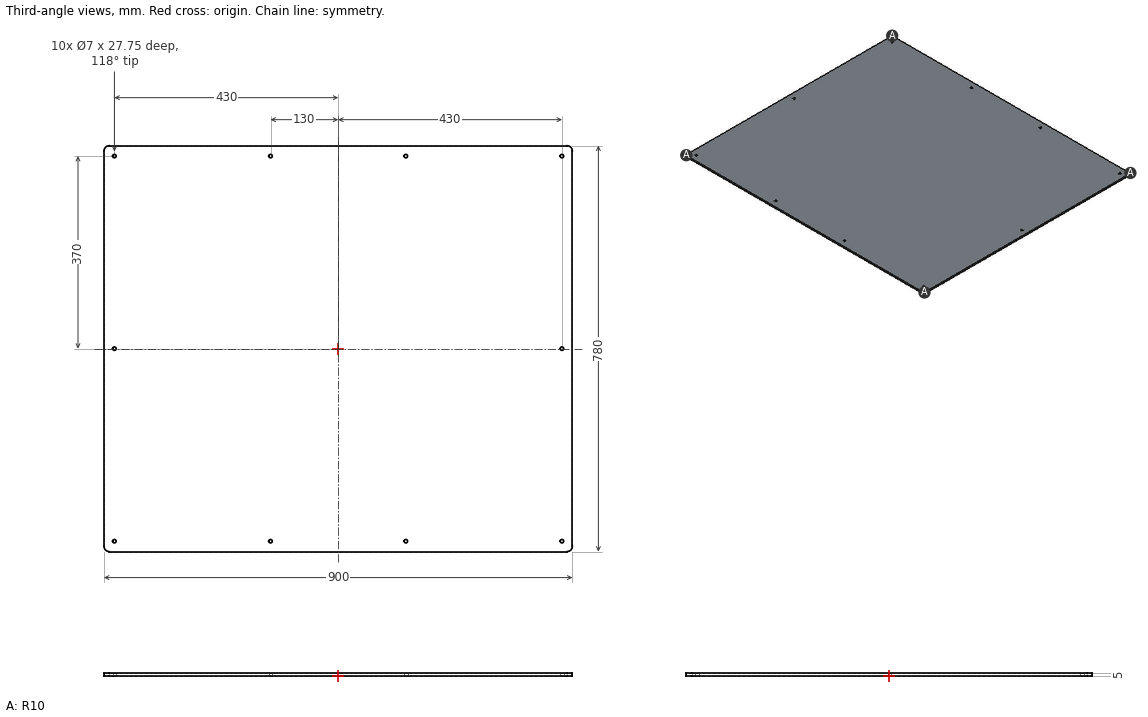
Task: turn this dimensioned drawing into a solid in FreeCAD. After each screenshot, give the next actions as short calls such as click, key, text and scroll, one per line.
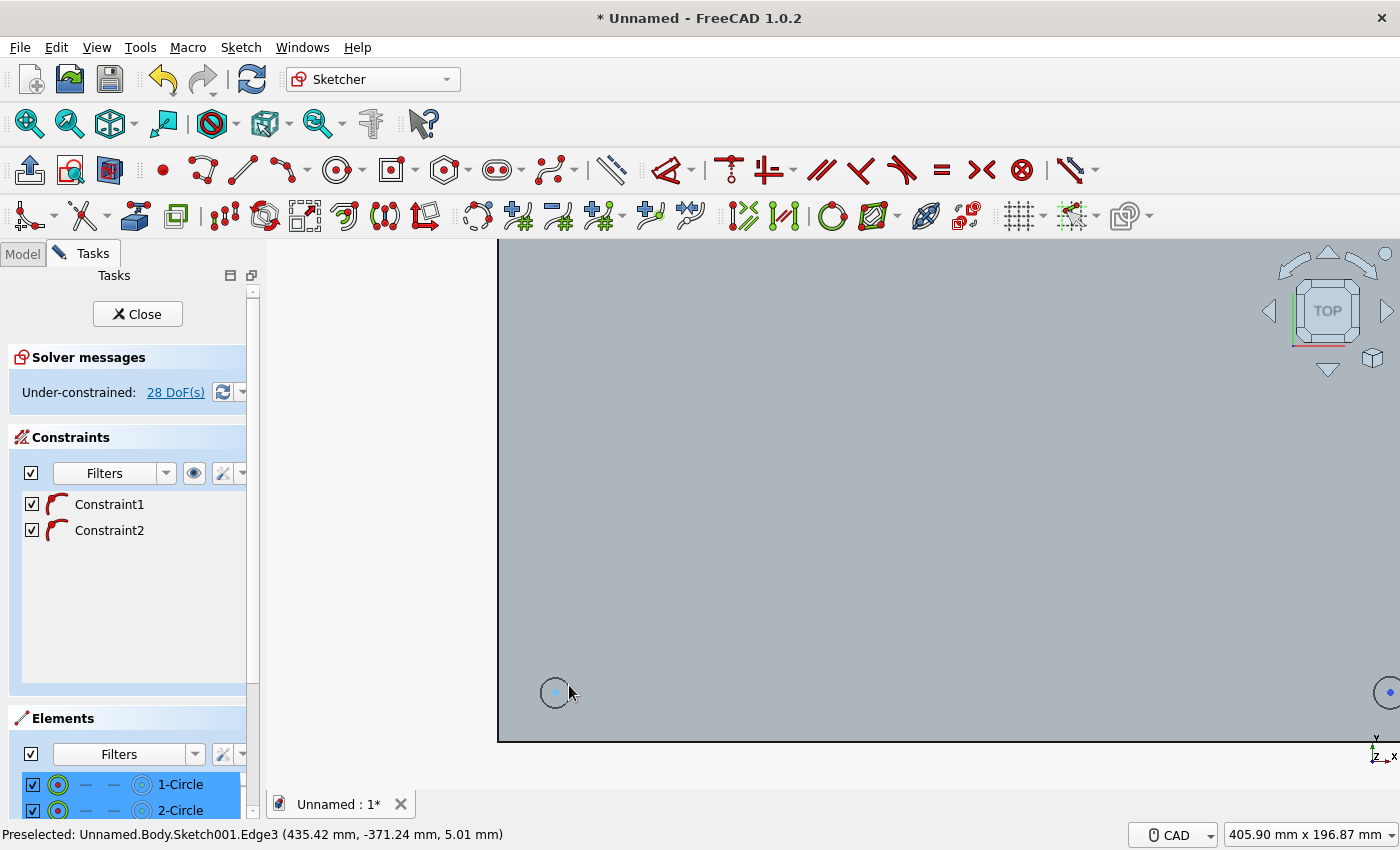
click(566, 682)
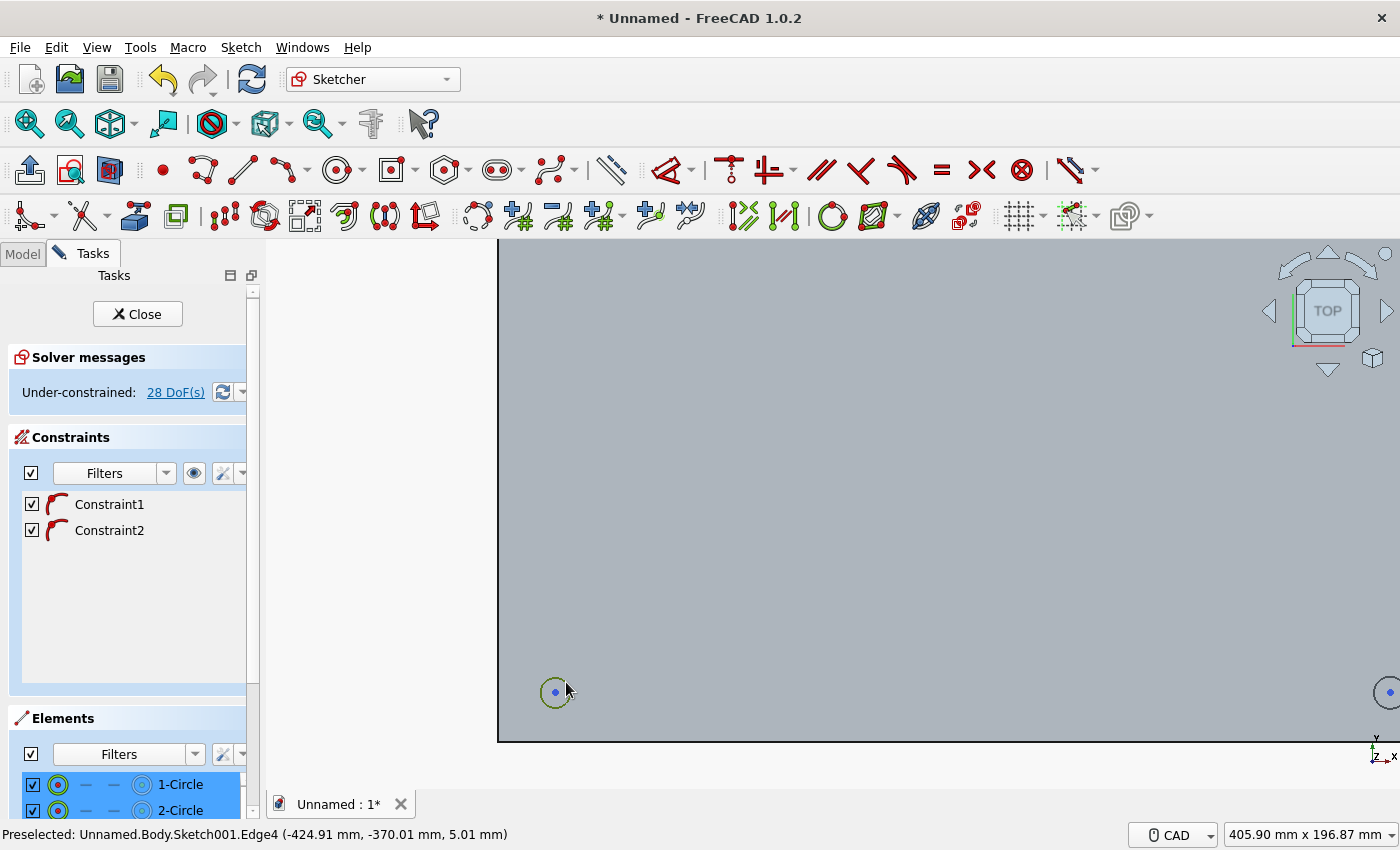
scroll(568, 685, down, 9)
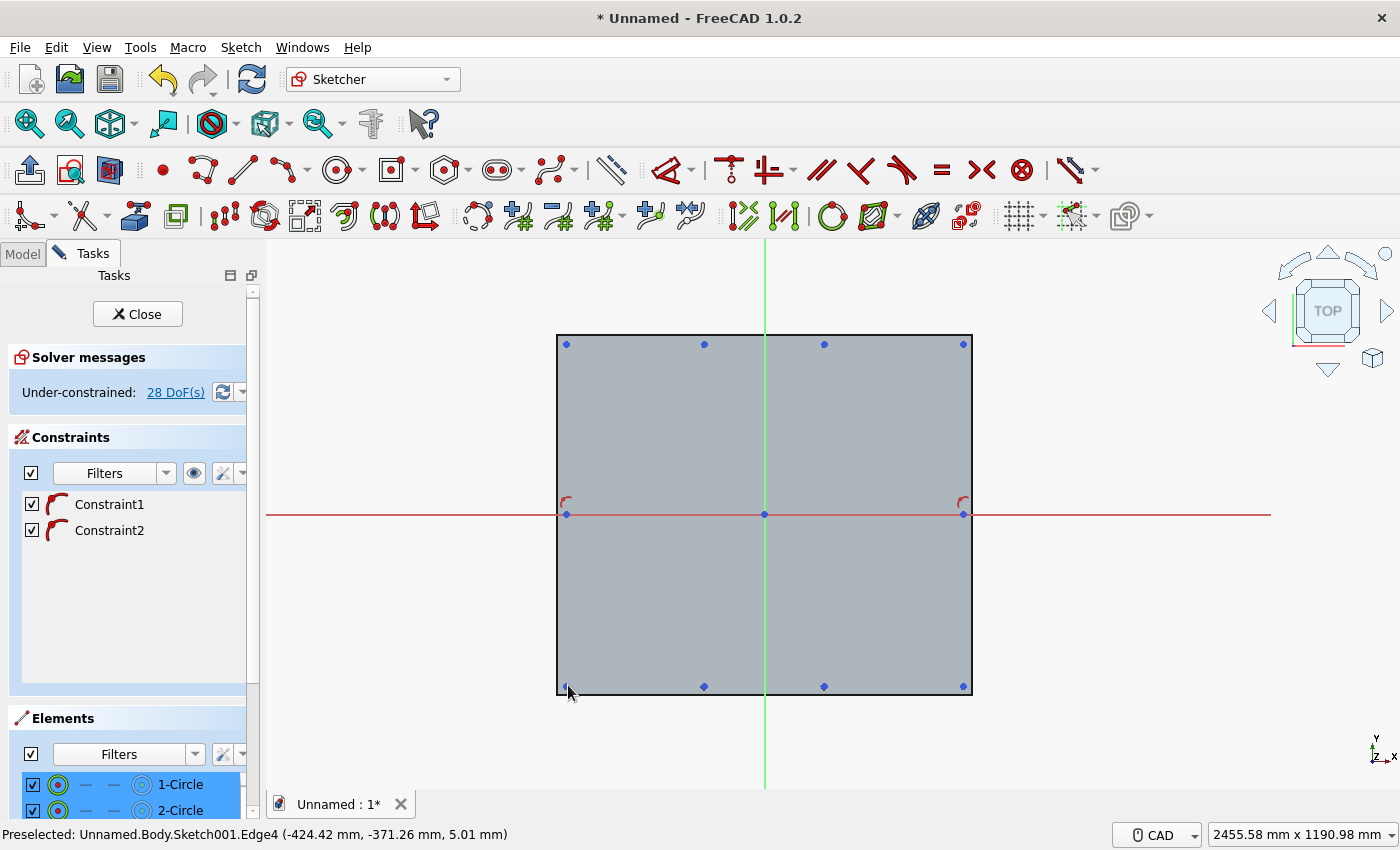
scroll(565, 515, up, 12)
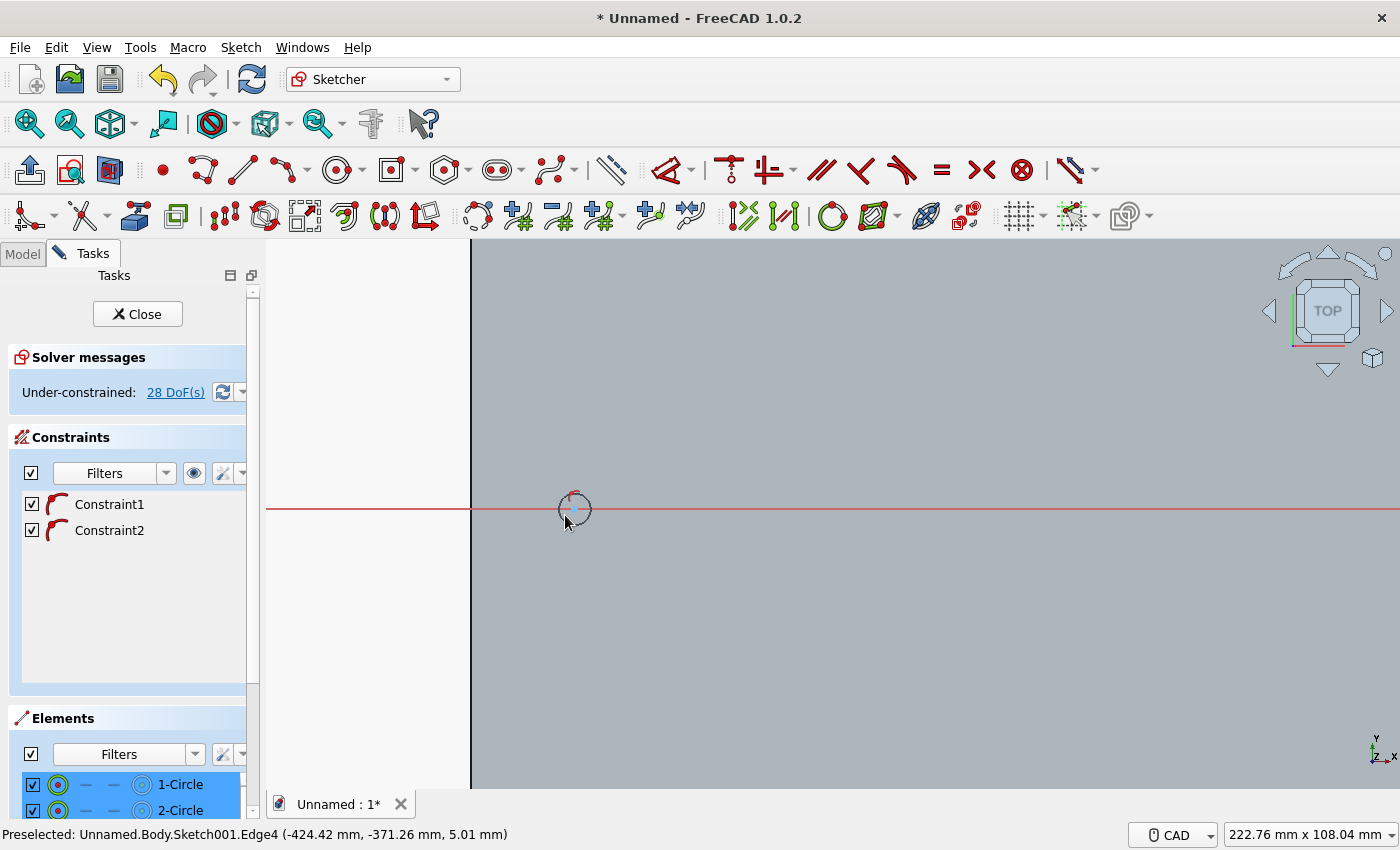
click(559, 509)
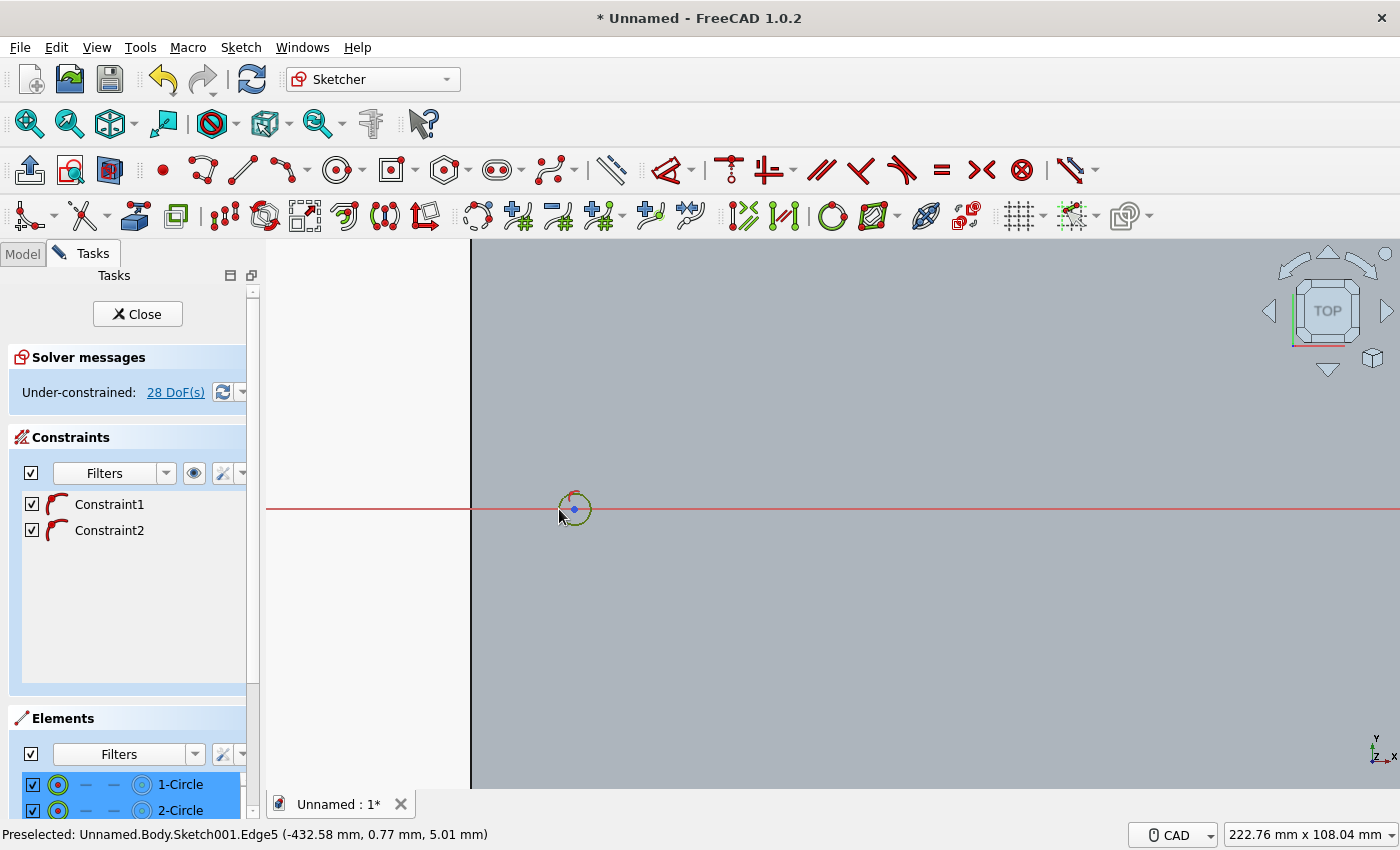
scroll(565, 514, down, 12)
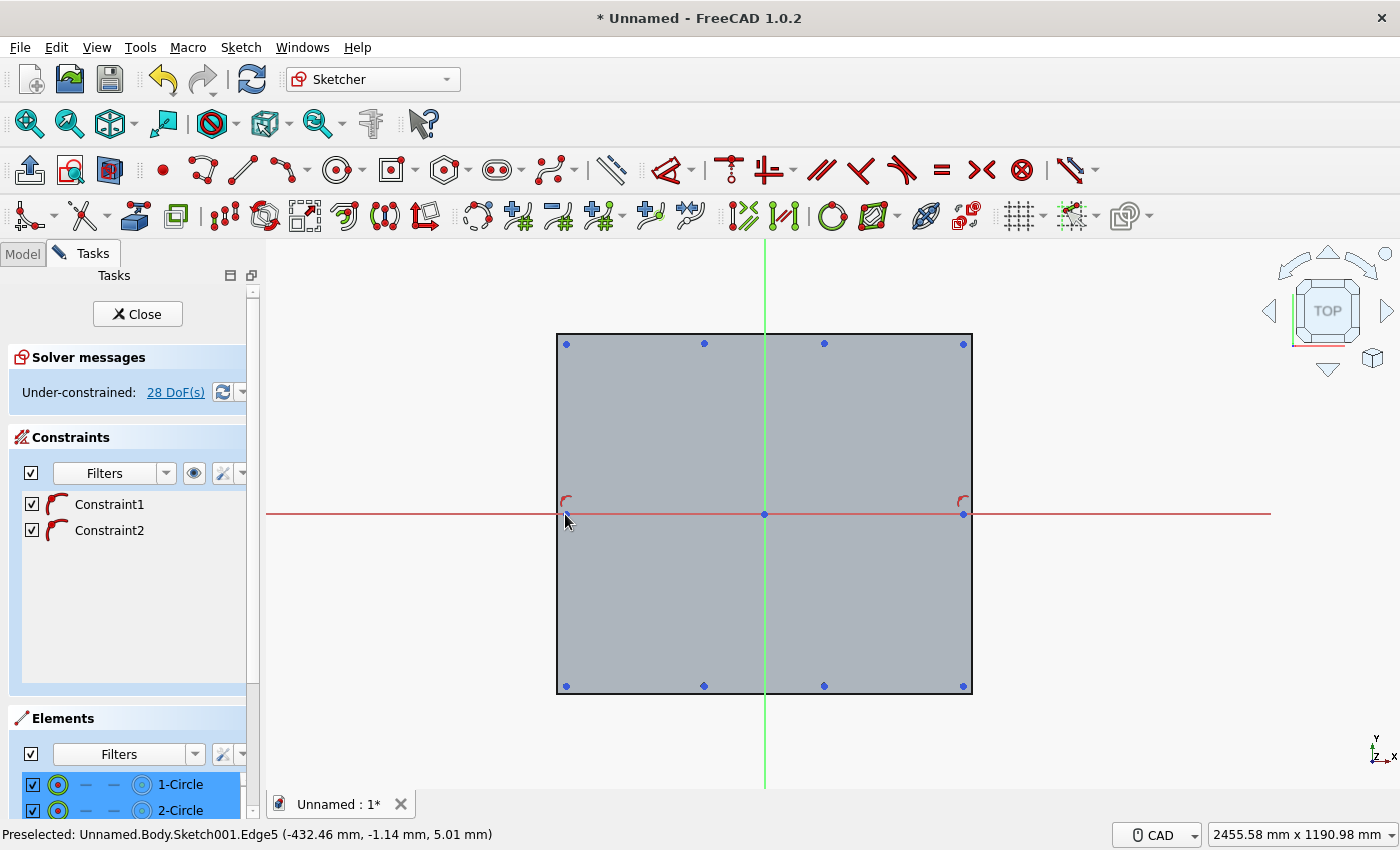
scroll(964, 513, up, 13)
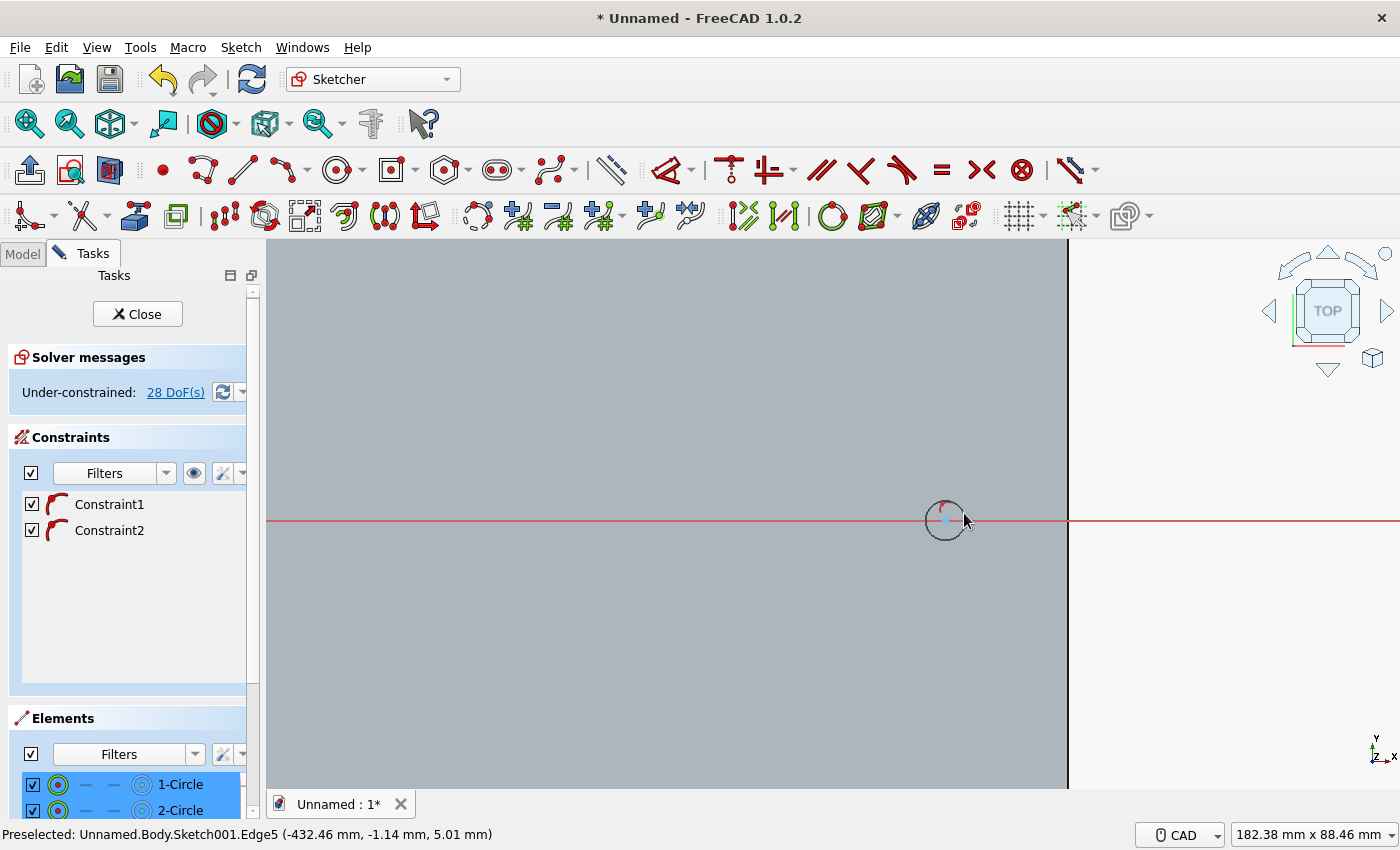
click(959, 507)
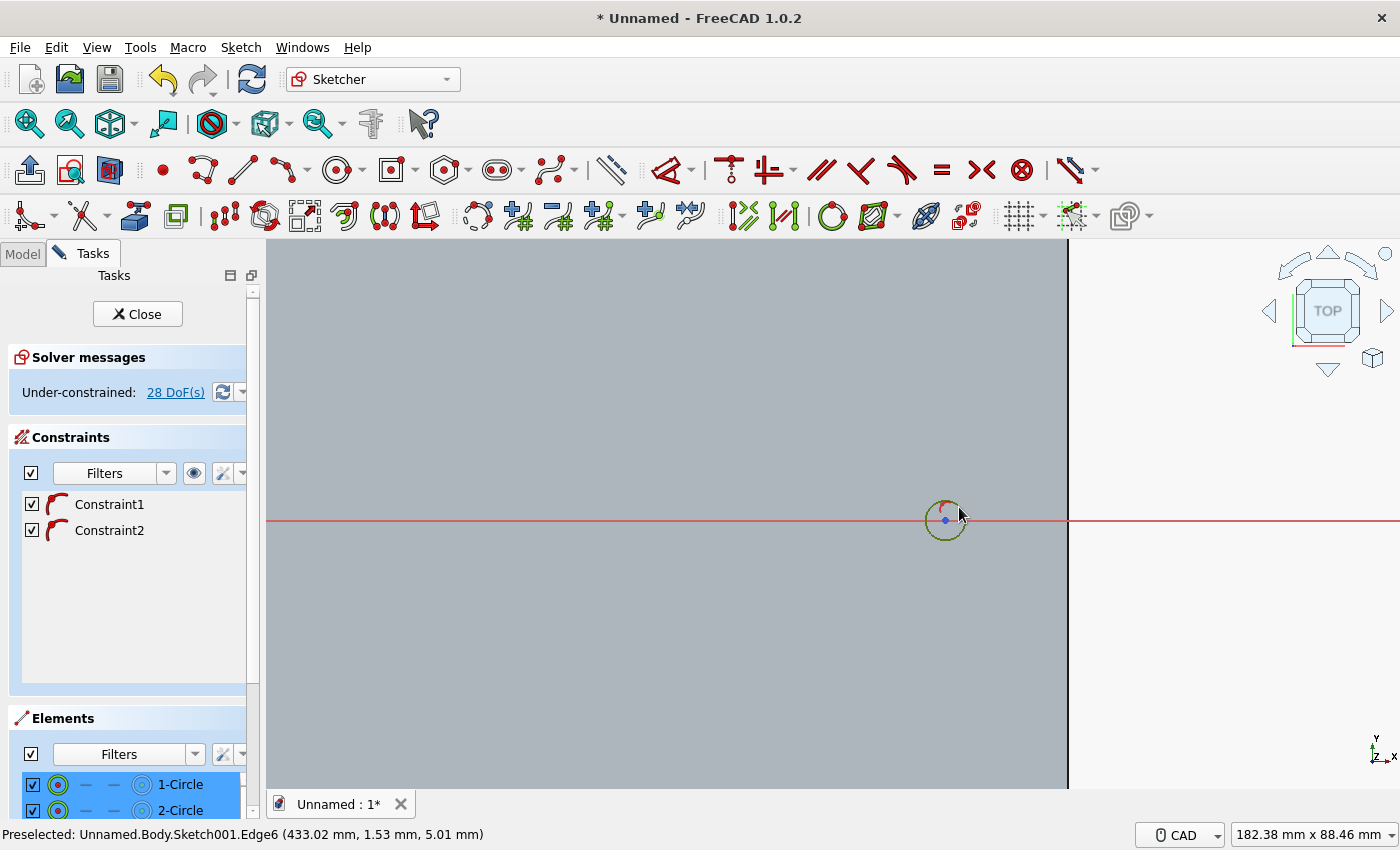
scroll(965, 513, down, 13)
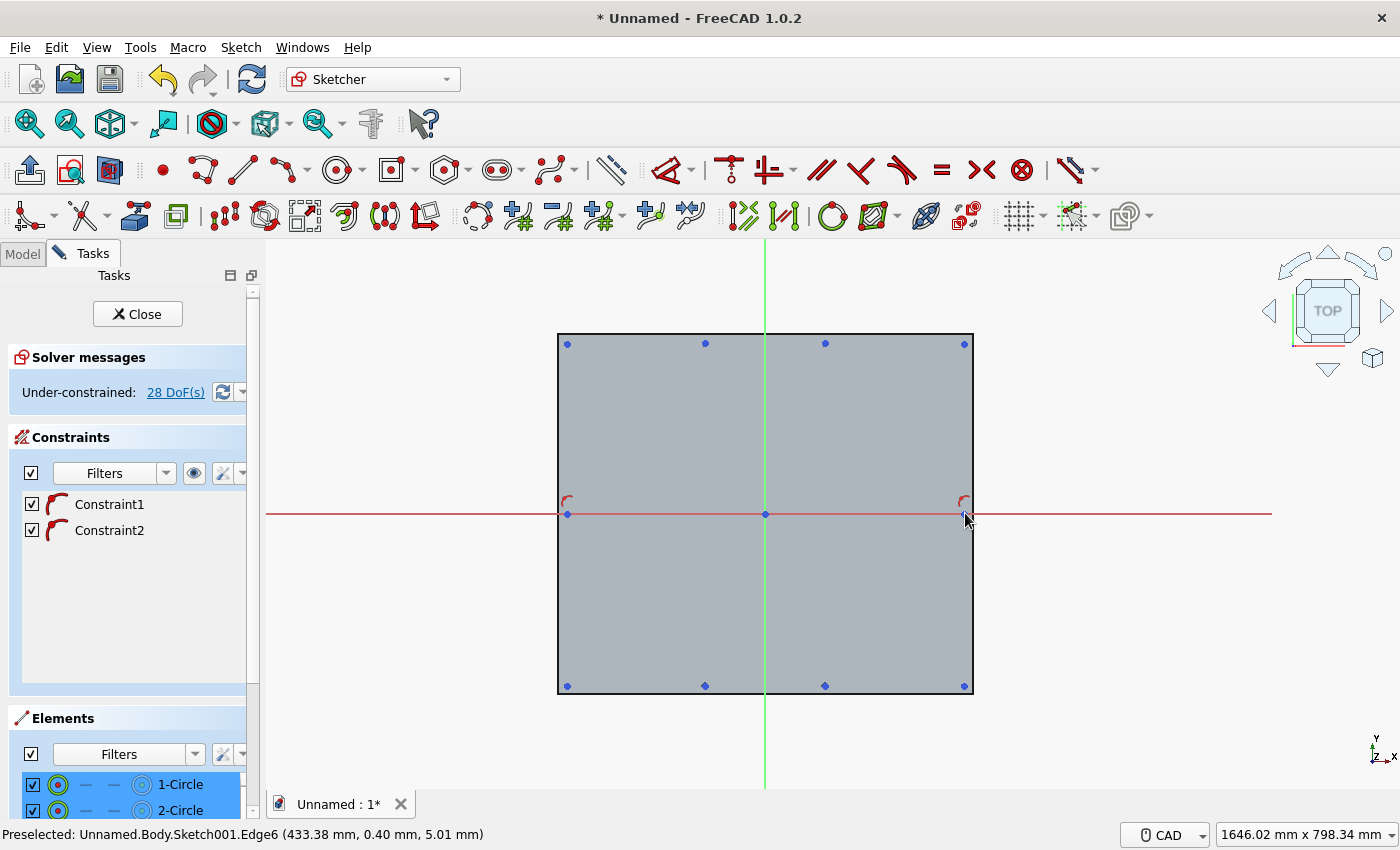
scroll(707, 342, up, 9)